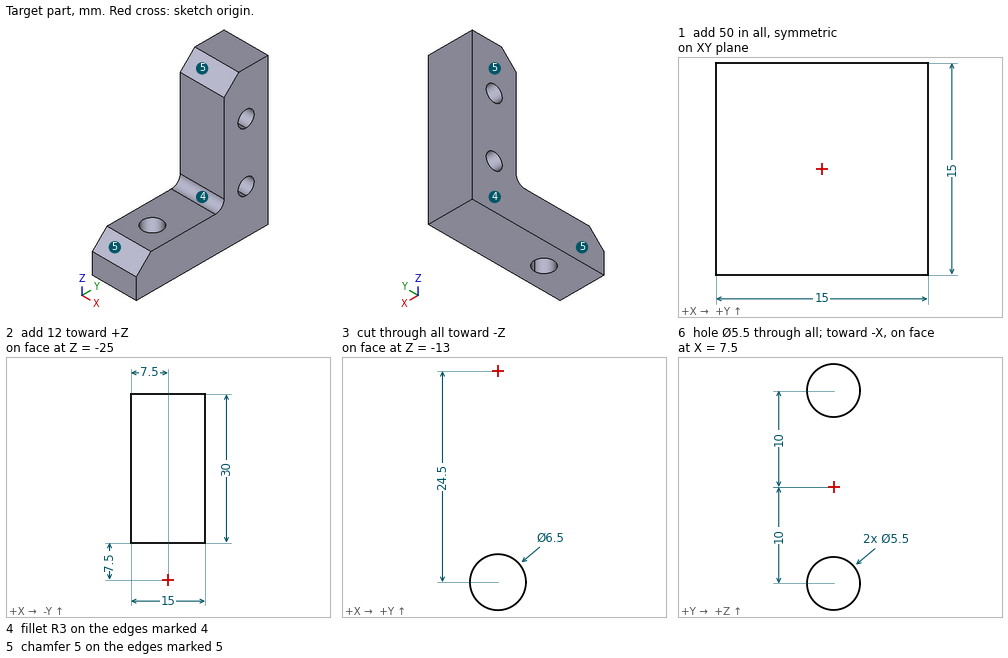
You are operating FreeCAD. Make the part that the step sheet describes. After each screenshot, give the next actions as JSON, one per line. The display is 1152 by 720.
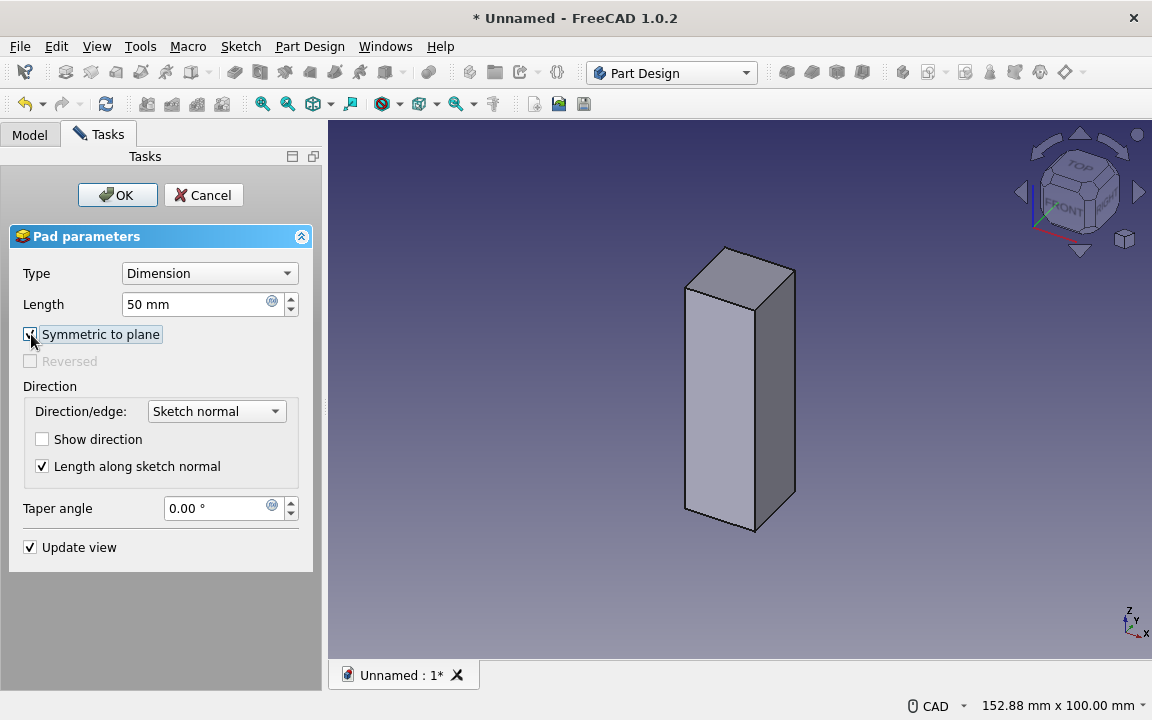
{"action": "left_click", "coordinate": [118, 195]}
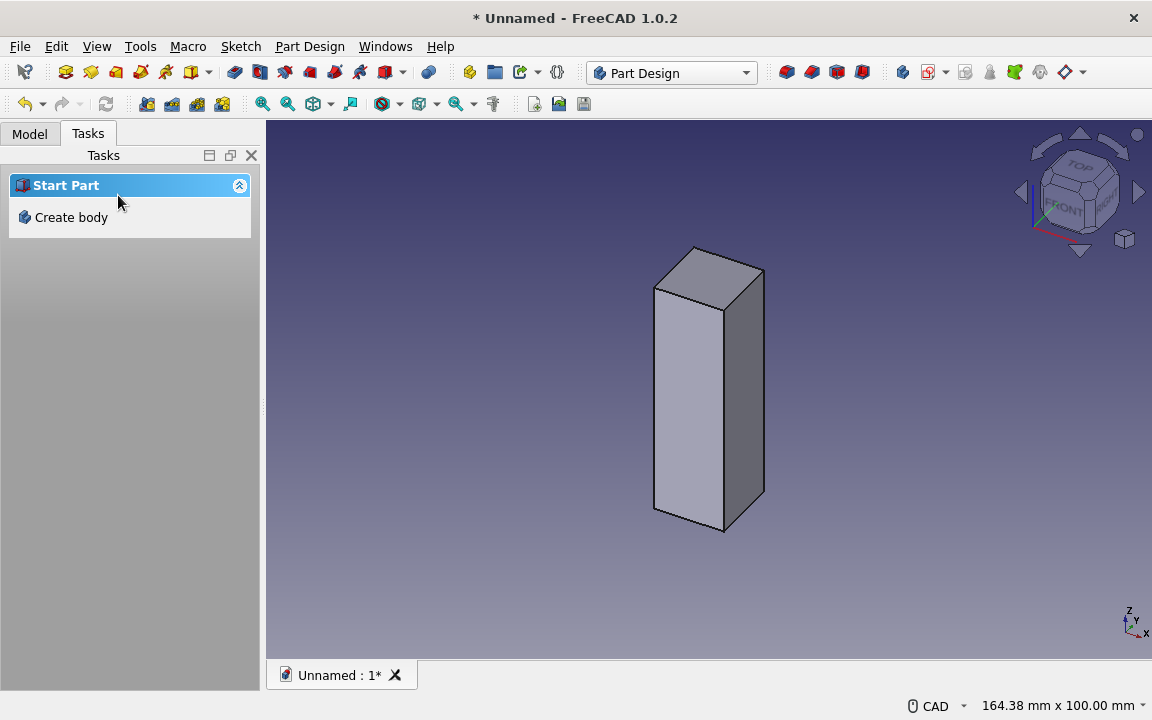
{"action": "key", "text": "5"}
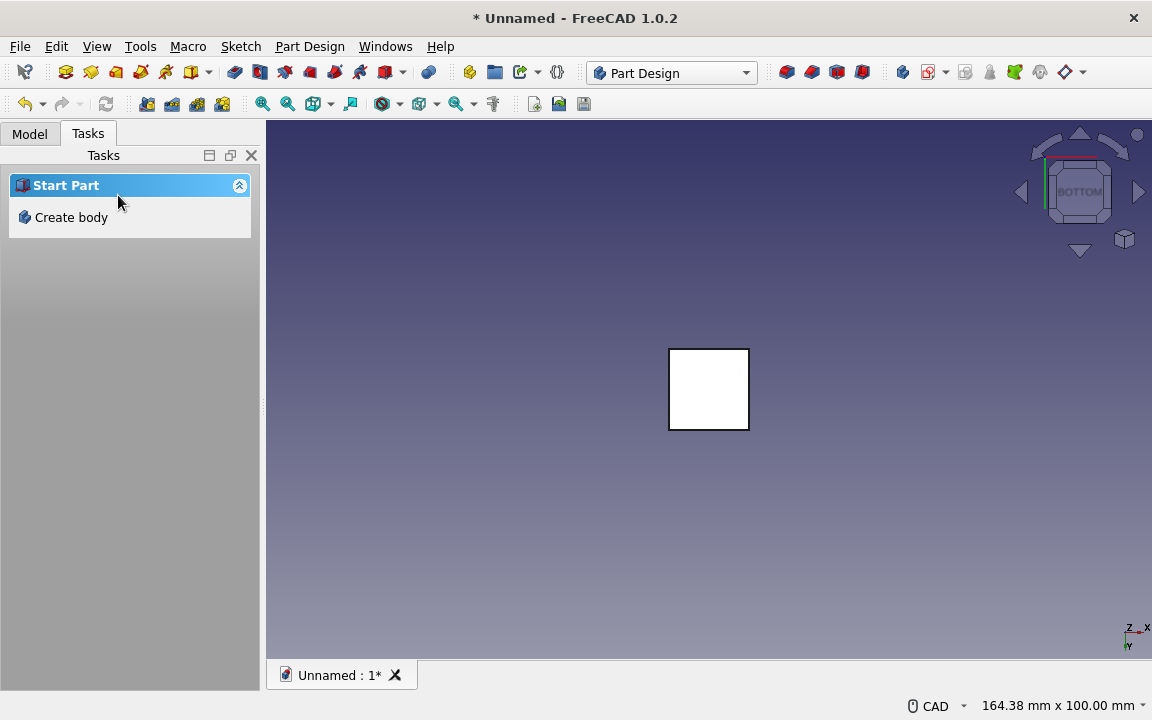
{"action": "left_click", "coordinate": [263, 104]}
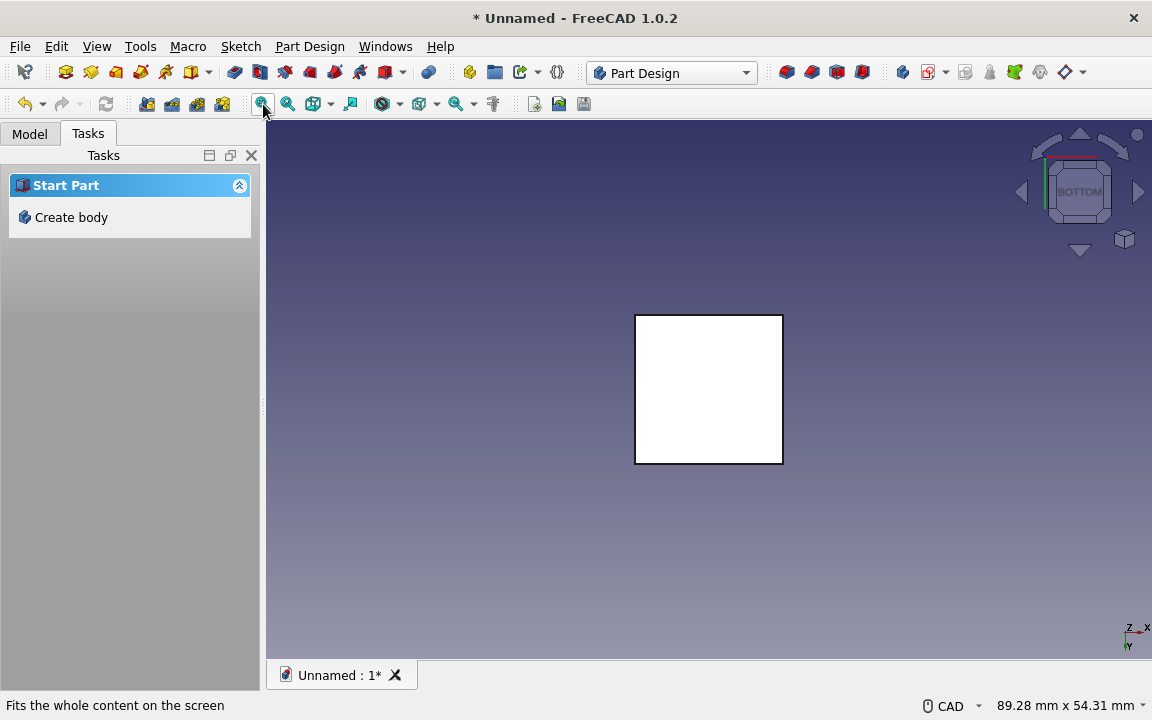
{"action": "left_click", "coordinate": [709, 388]}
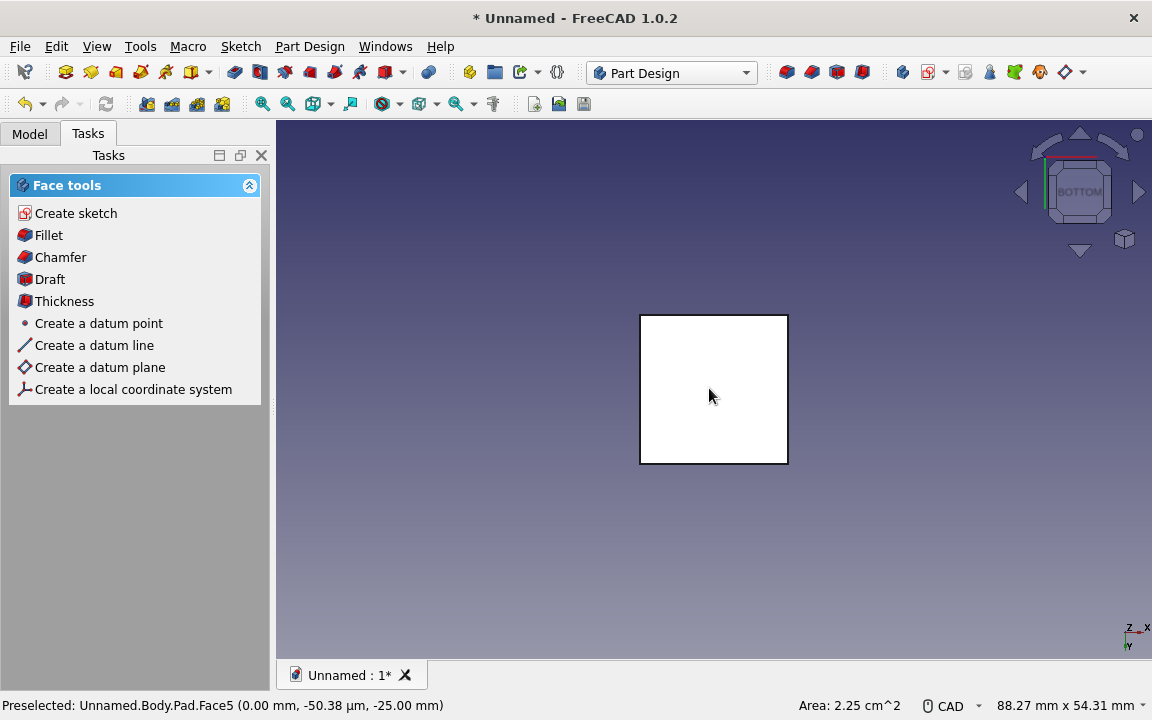
{"action": "left_click", "coordinate": [928, 72]}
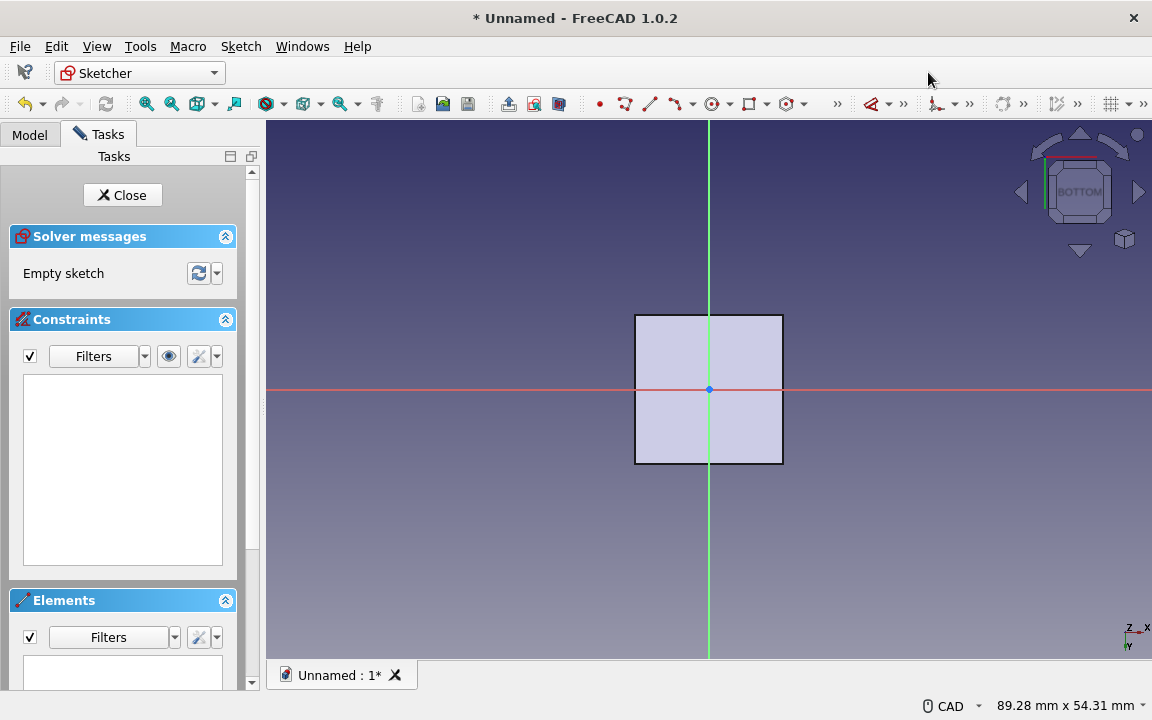
{"action": "scroll", "coordinate": [501, 631], "scroll_direction": "down", "scroll_amount": 2}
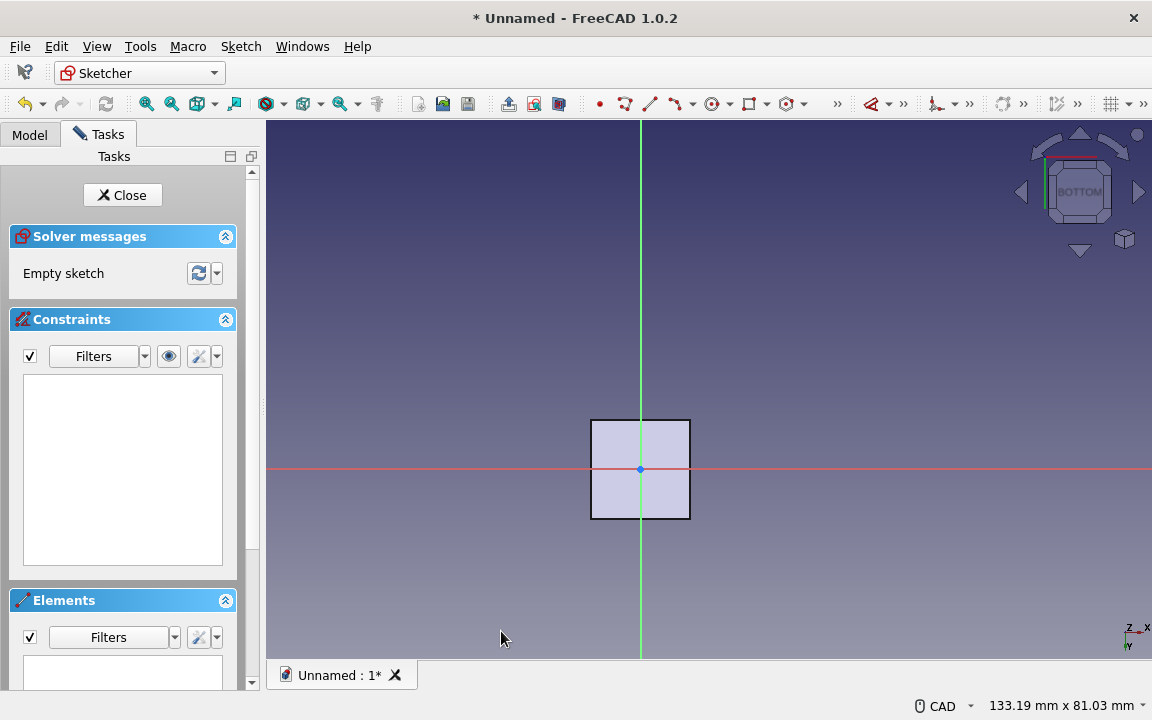
{"action": "scroll", "coordinate": [641, 254], "scroll_direction": "up", "scroll_amount": 2}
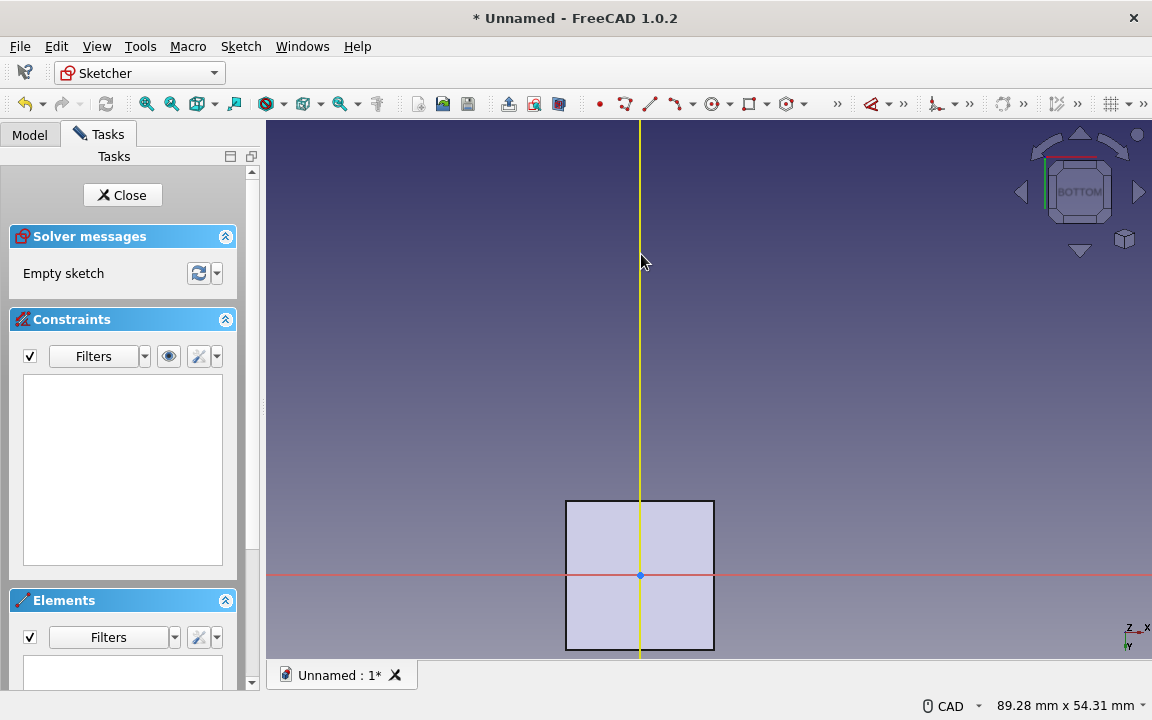
{"action": "key", "text": "g r"}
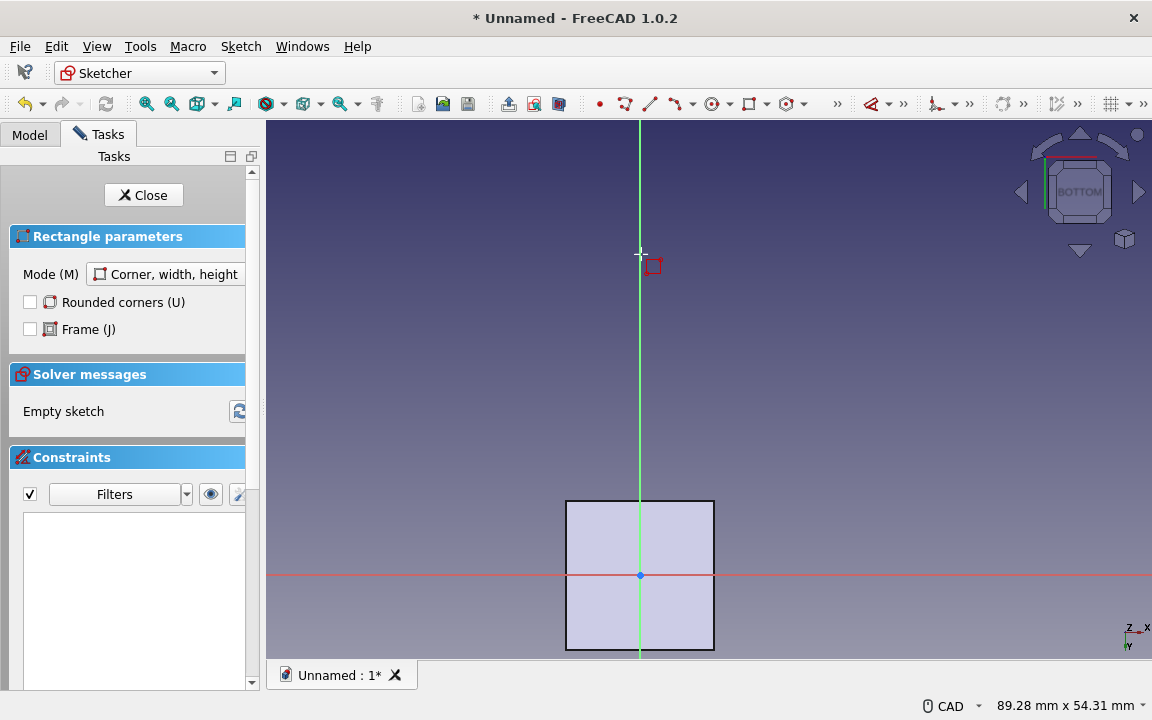
{"action": "left_click", "coordinate": [566, 203]}
{"action": "mouse_move", "coordinate": [714, 501]}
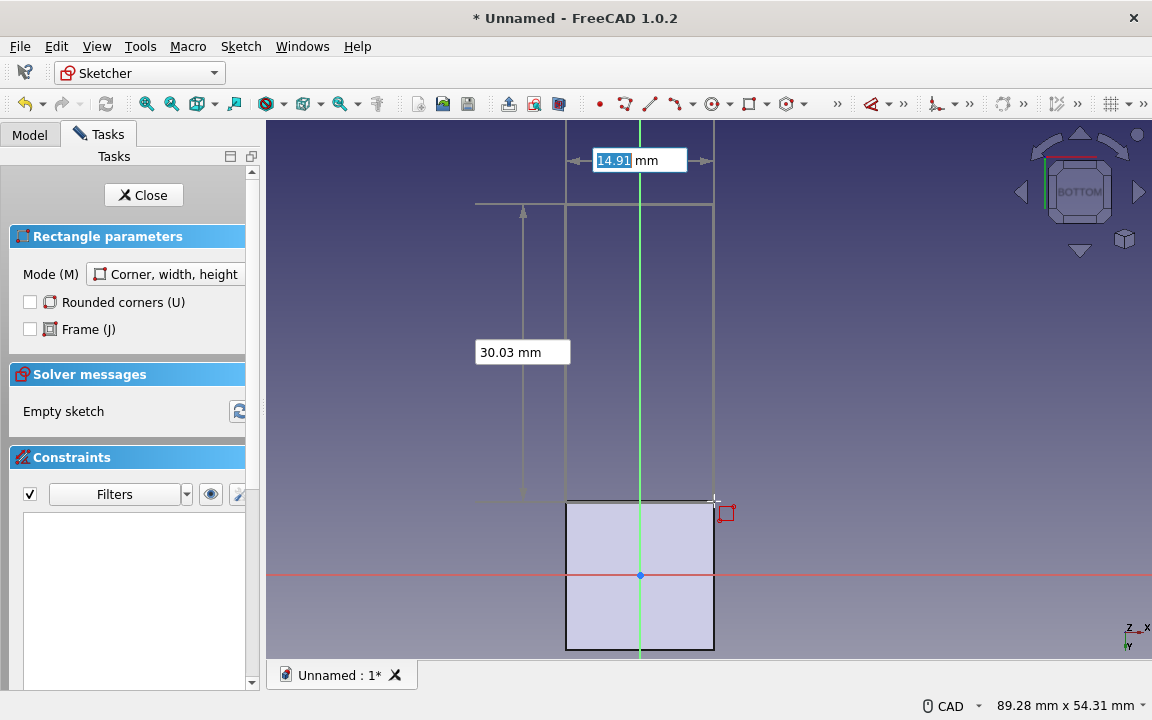
{"action": "type", "text": "15"}
{"action": "key", "text": "Tab"}
{"action": "type", "text": "30"}
{"action": "key", "text": "Return"}
{"action": "key", "text": "Escape"}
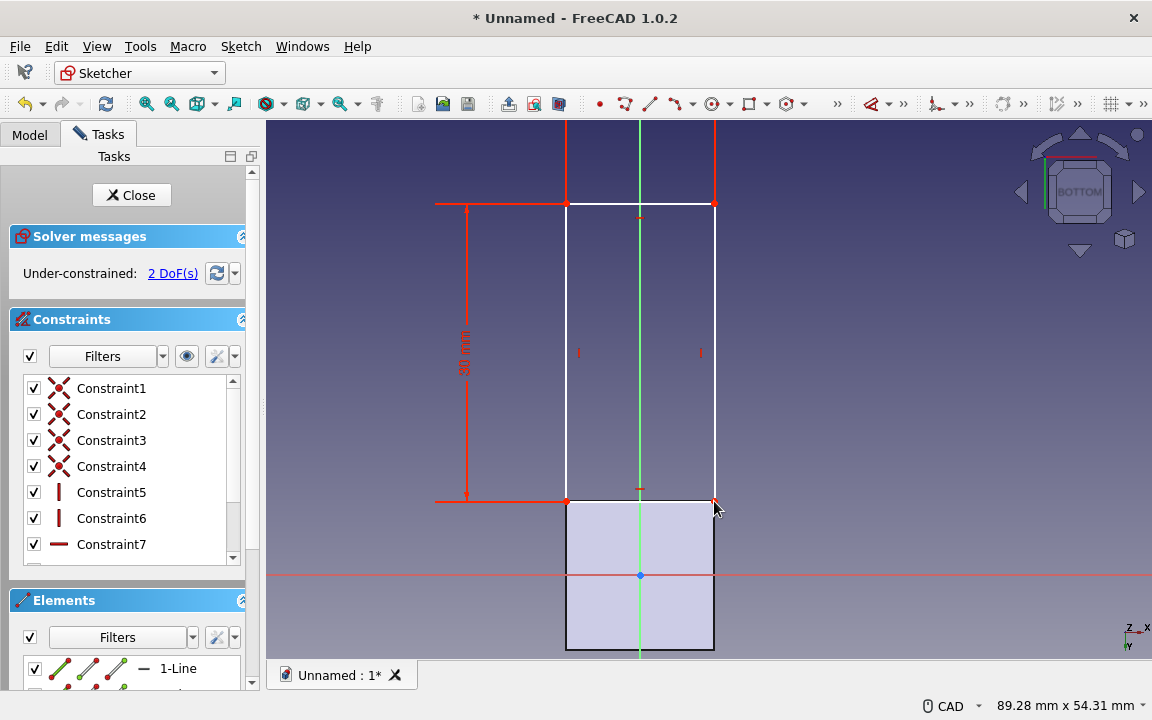
{"action": "left_click", "coordinate": [566, 204]}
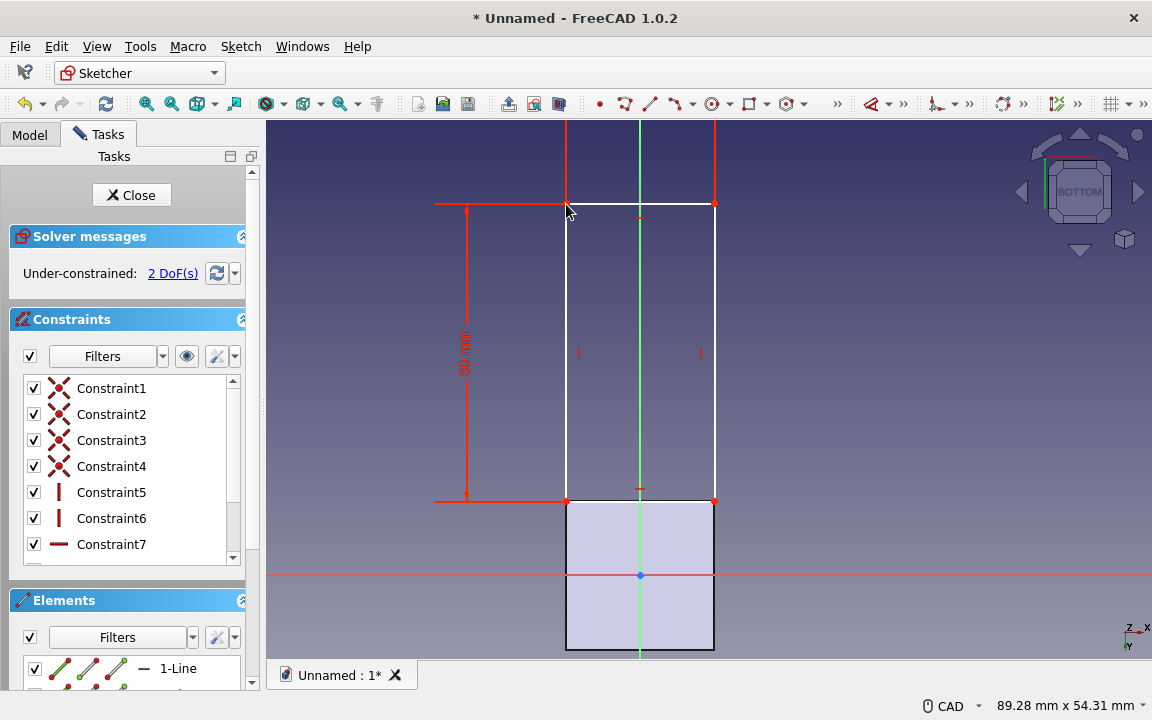
{"action": "key", "text": "l"}